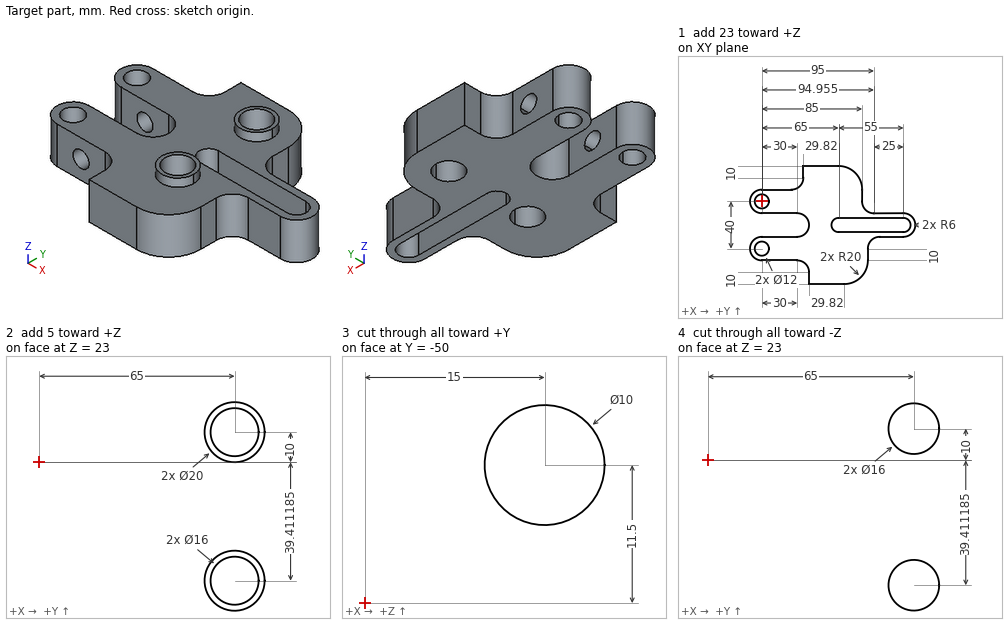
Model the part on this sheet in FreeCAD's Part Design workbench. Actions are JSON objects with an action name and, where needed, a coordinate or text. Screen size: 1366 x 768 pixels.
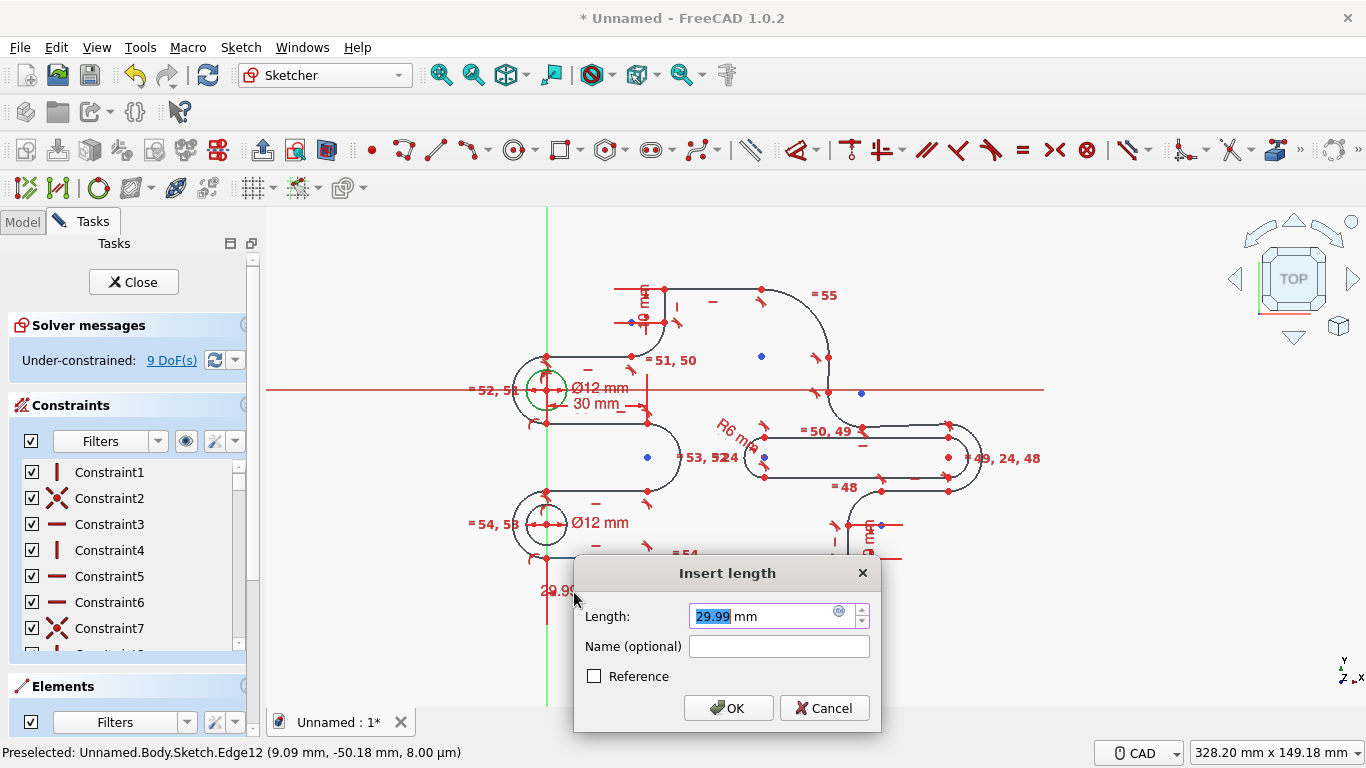
{"action": "type", "text": "30"}
{"action": "key", "text": "Return"}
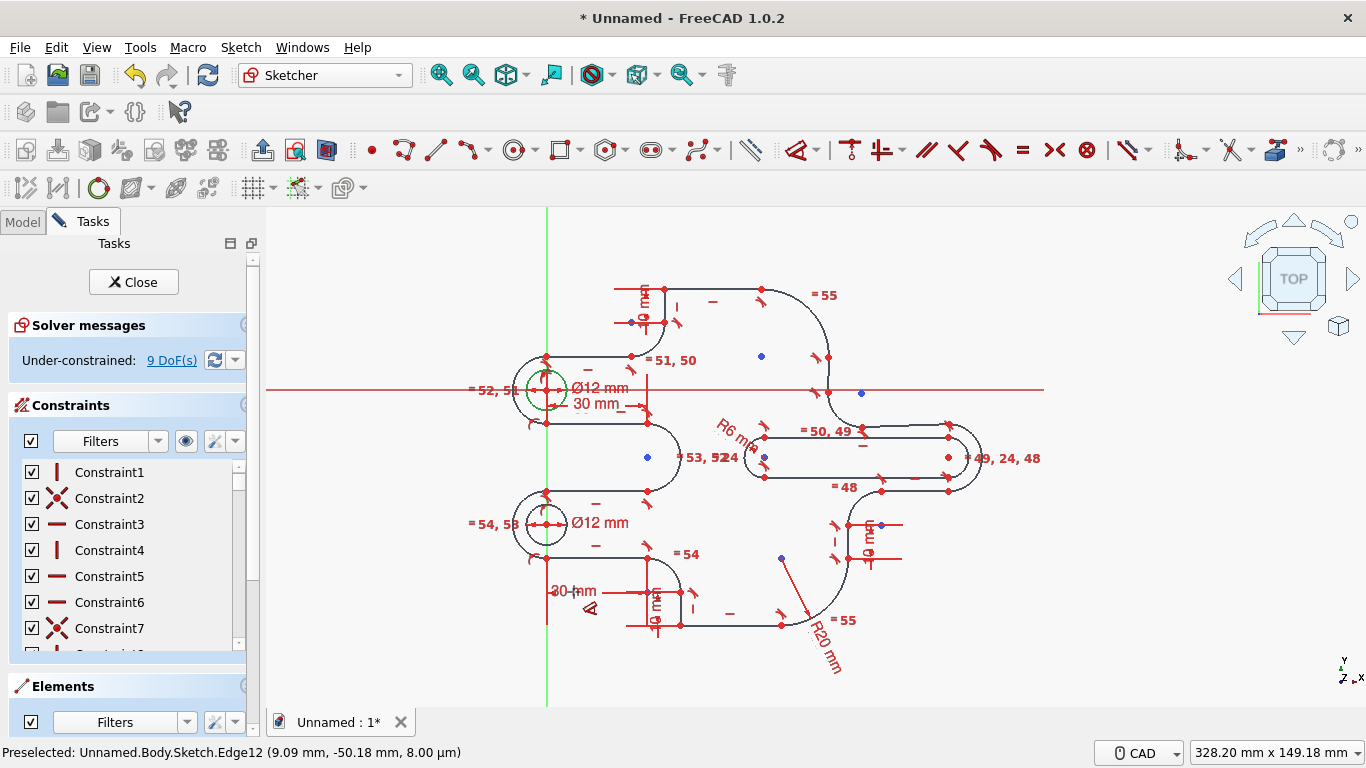
{"action": "left_click", "coordinate": [820, 438]}
{"action": "left_click", "coordinate": [856, 404]}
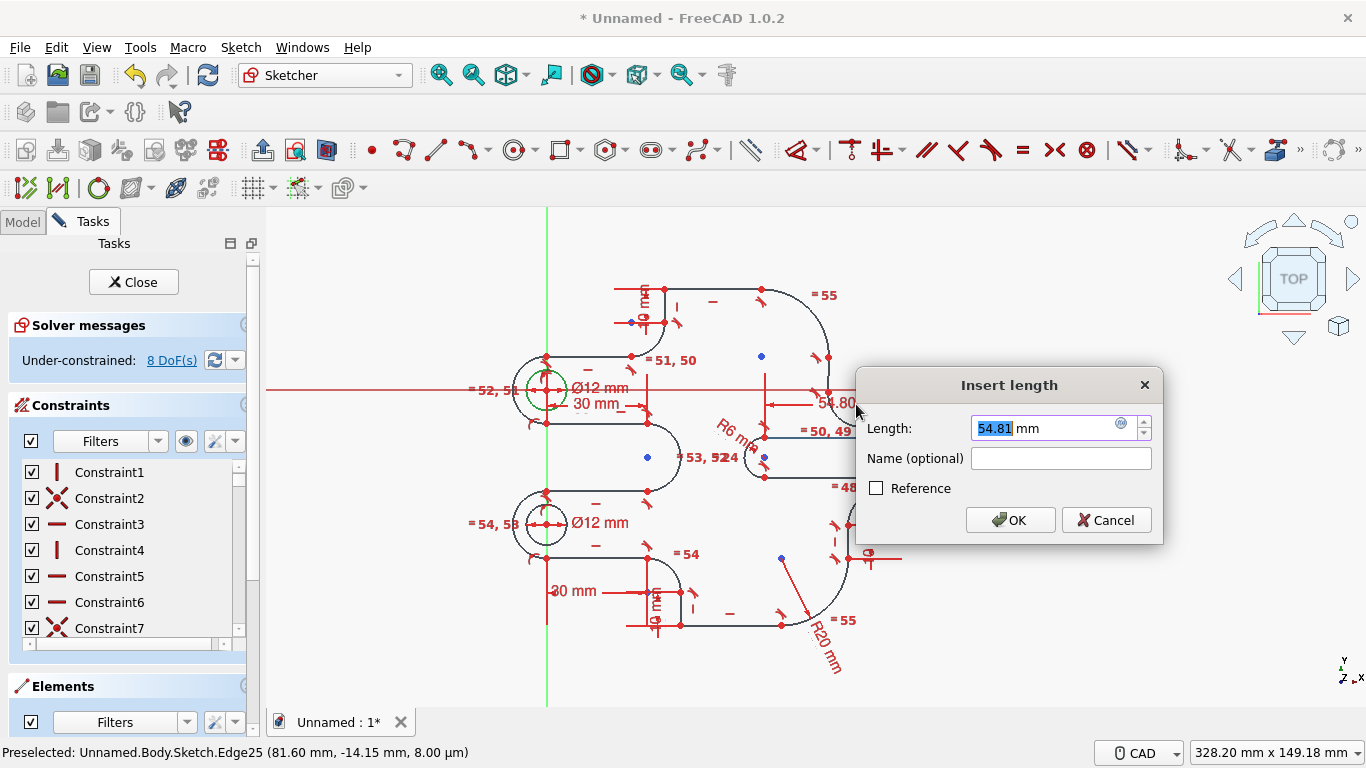
{"action": "type", "text": "55"}
{"action": "key", "text": "Return"}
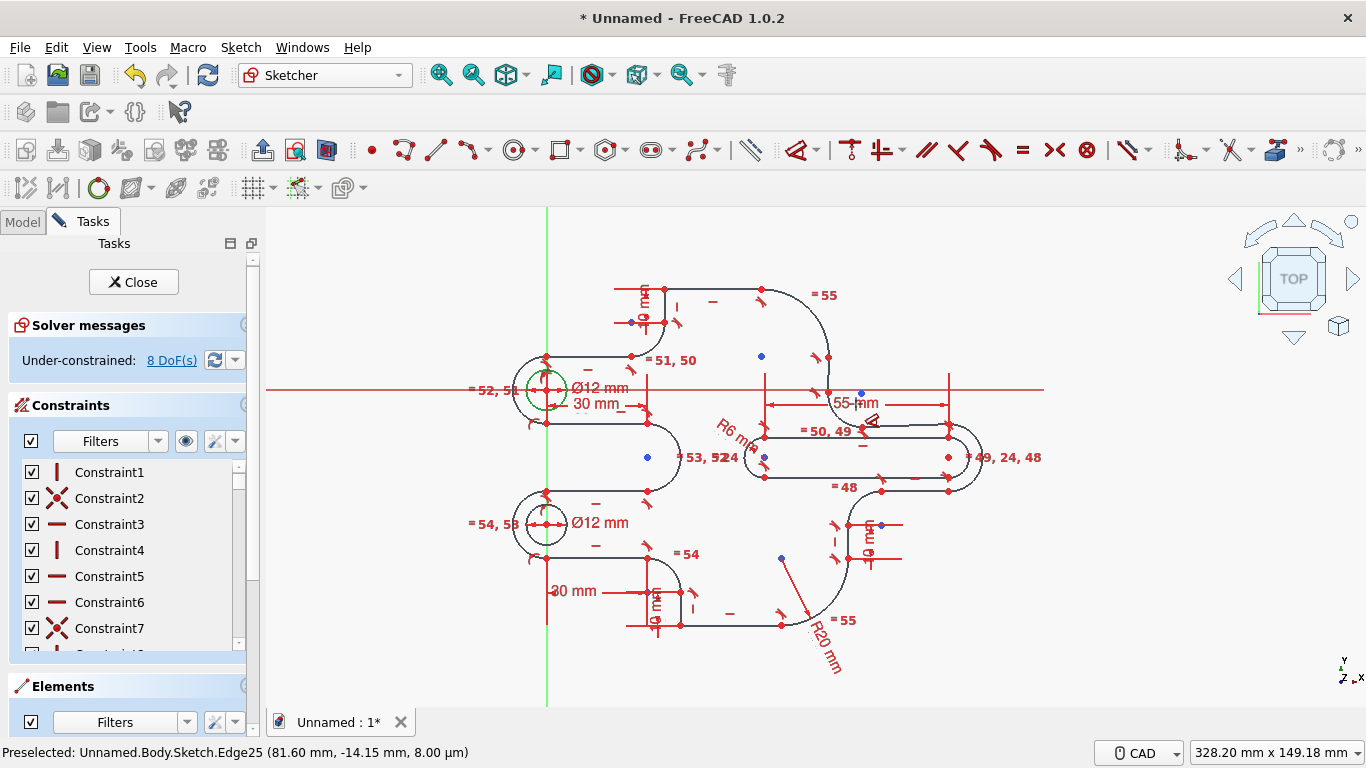
{"action": "left_click", "coordinate": [547, 525]}
{"action": "left_click", "coordinate": [513, 458]}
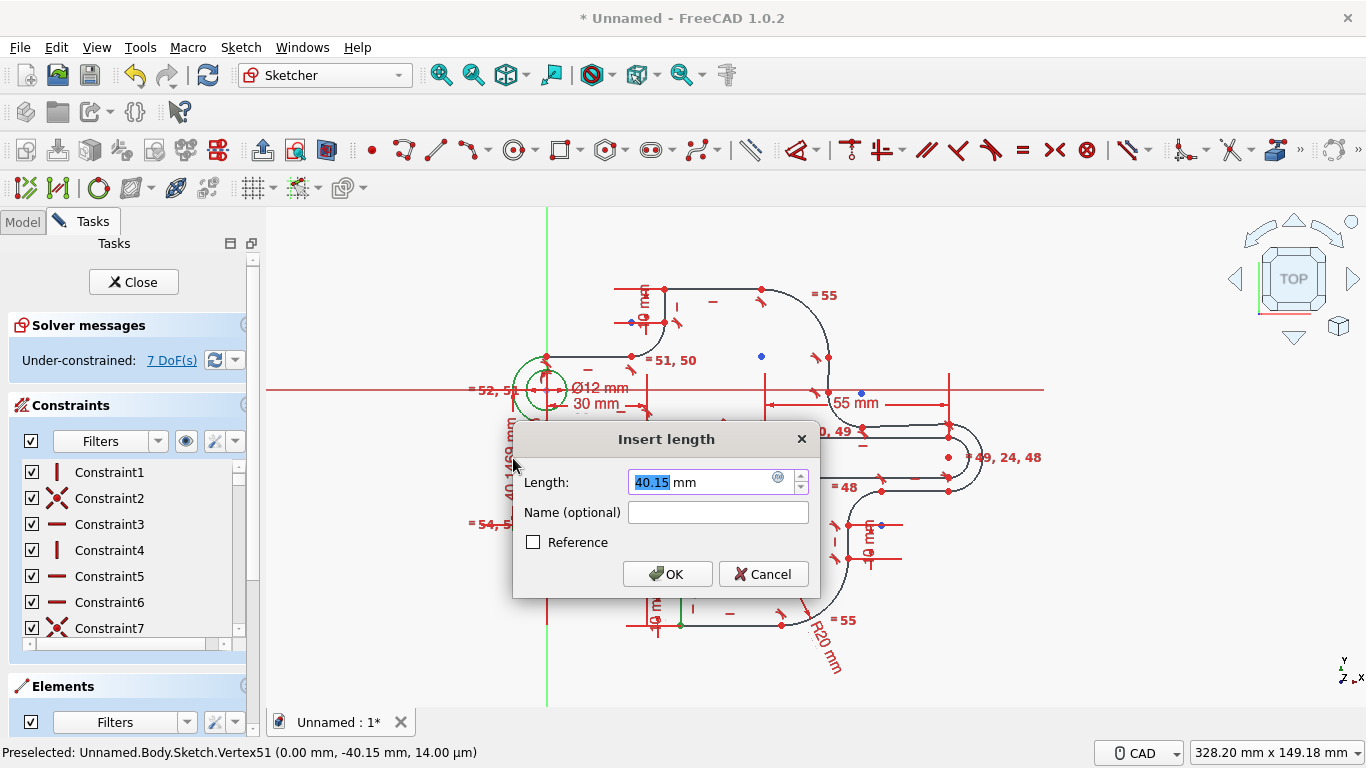
{"action": "type", "text": "40"}
{"action": "key", "text": "Return"}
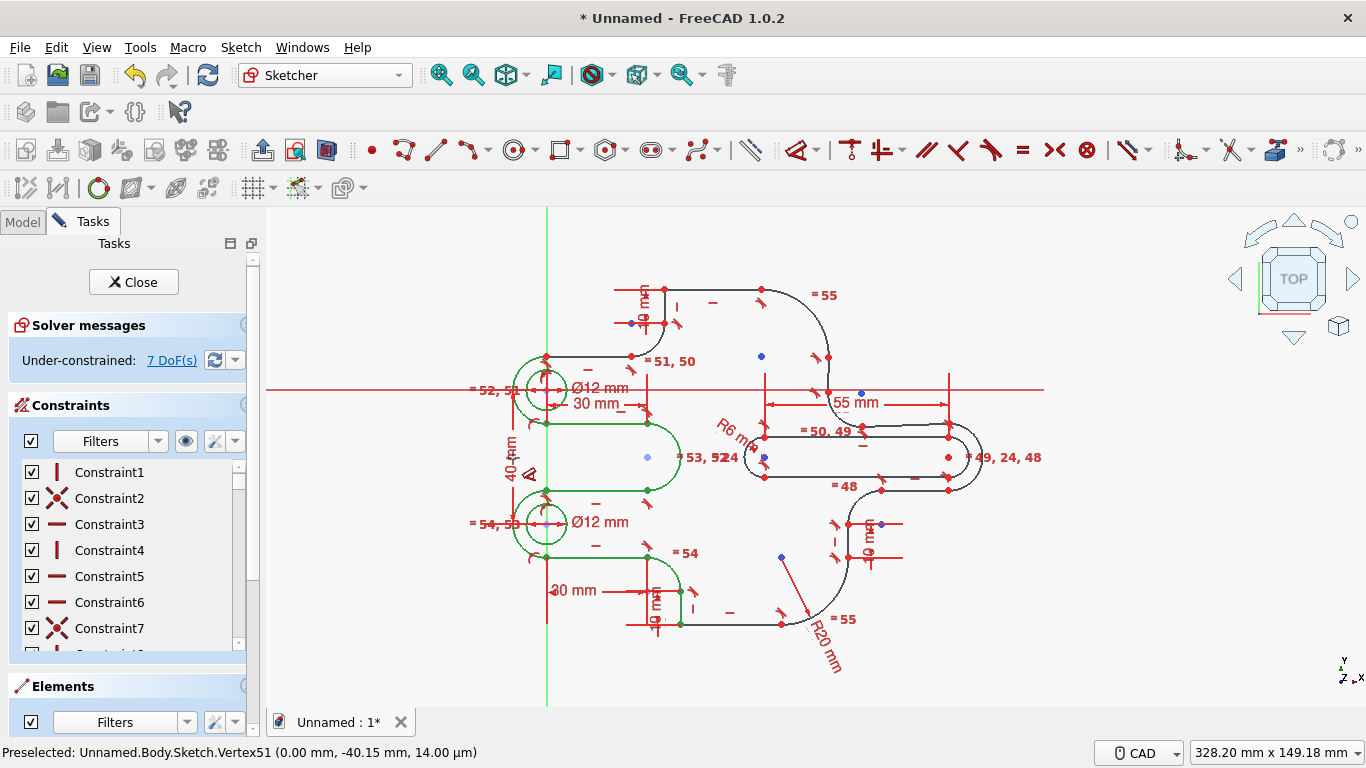
{"action": "left_click", "coordinate": [863, 427]}
{"action": "left_click", "coordinate": [705, 356]}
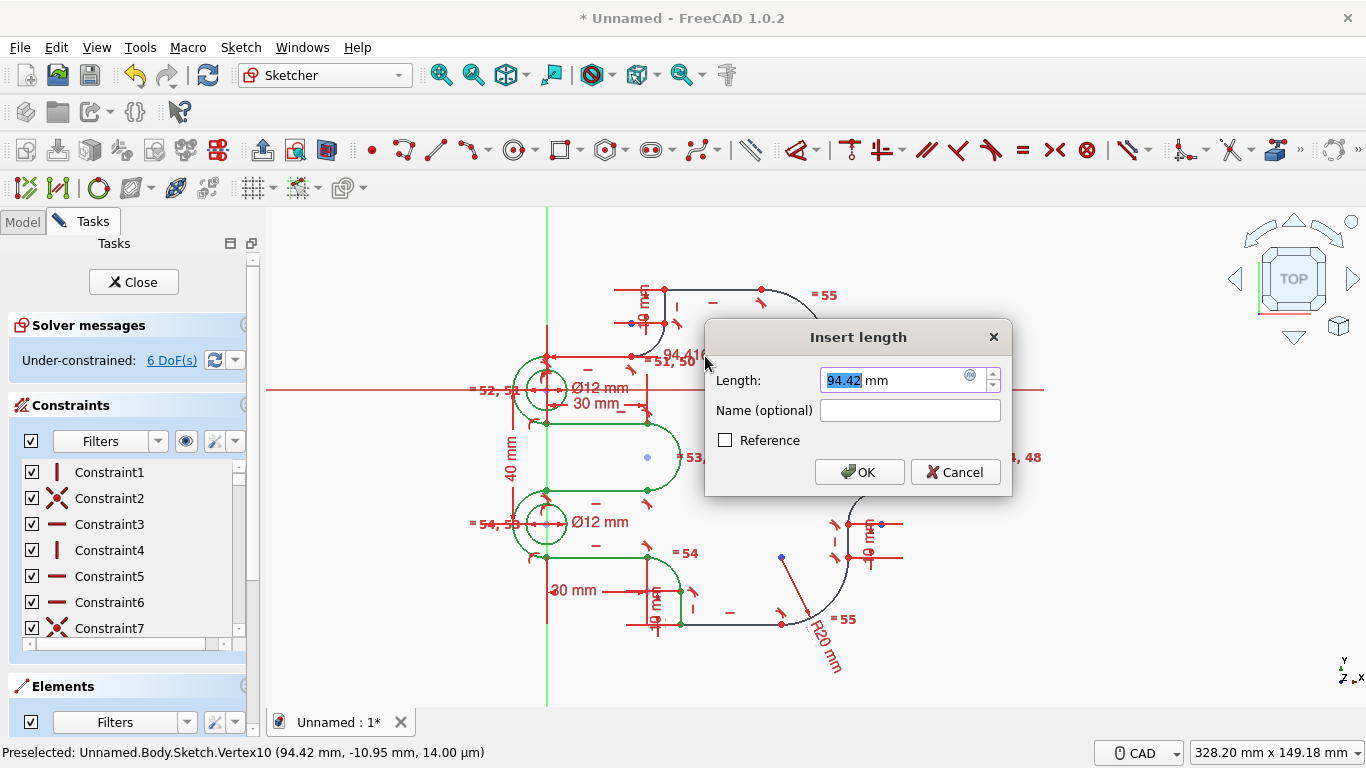
{"action": "type", "text": "95"}
{"action": "key", "text": "Return"}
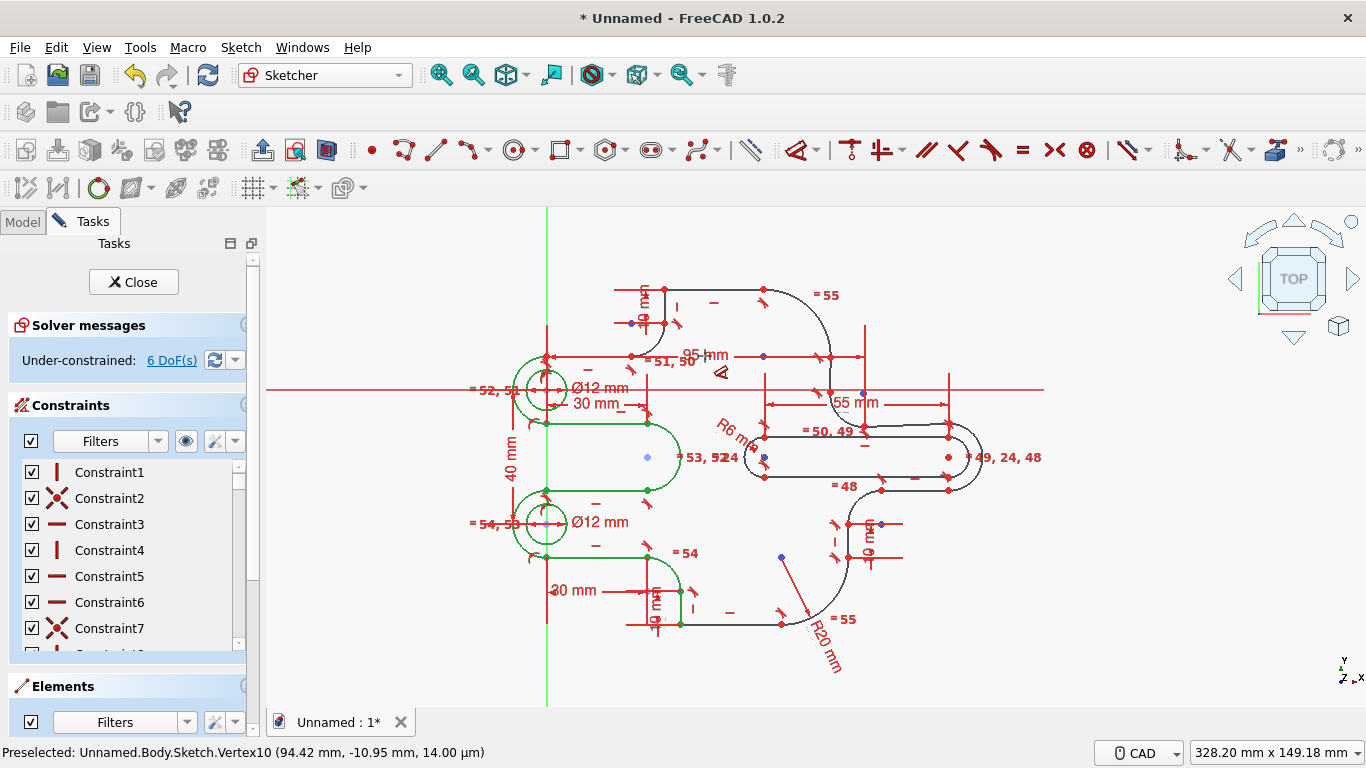
{"action": "left_click", "coordinate": [831, 358]}
{"action": "left_click", "coordinate": [754, 324]}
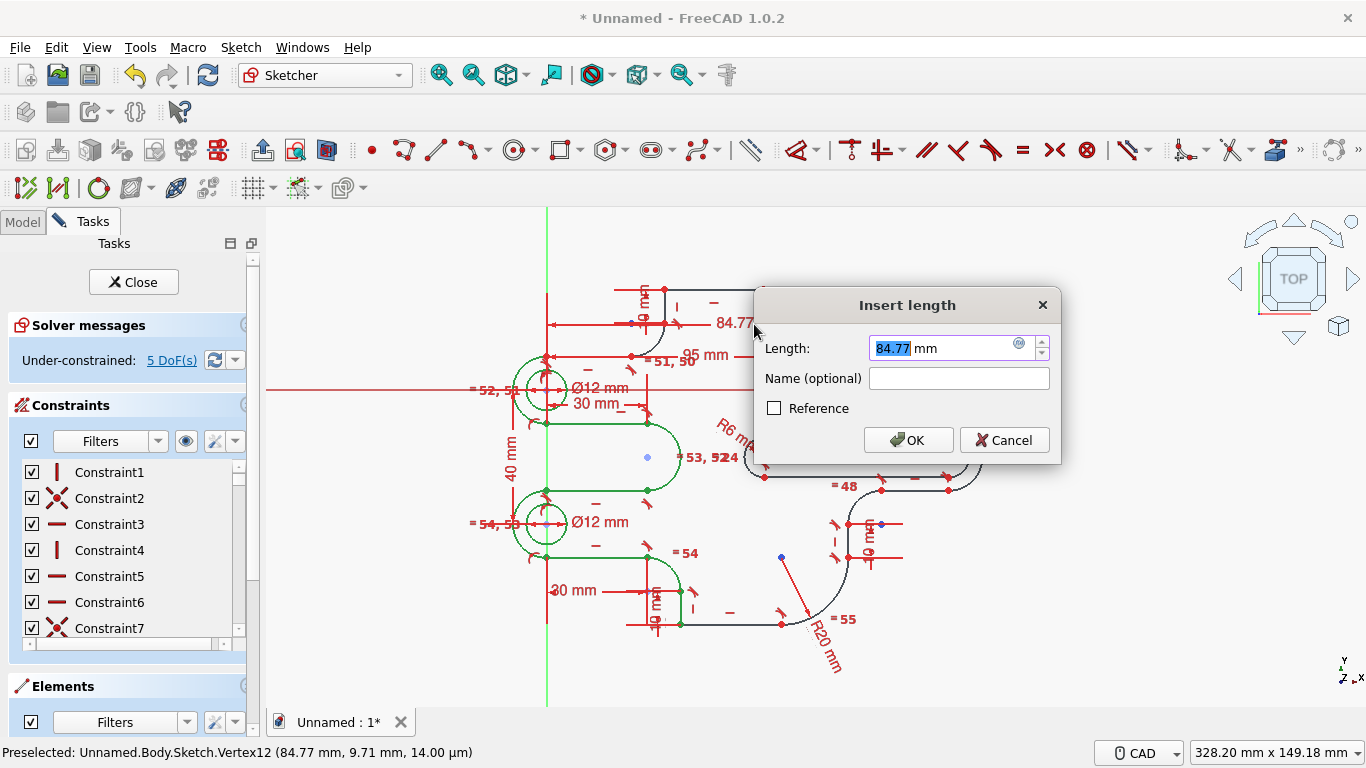
{"action": "type", "text": "85"}
{"action": "key", "text": "Return"}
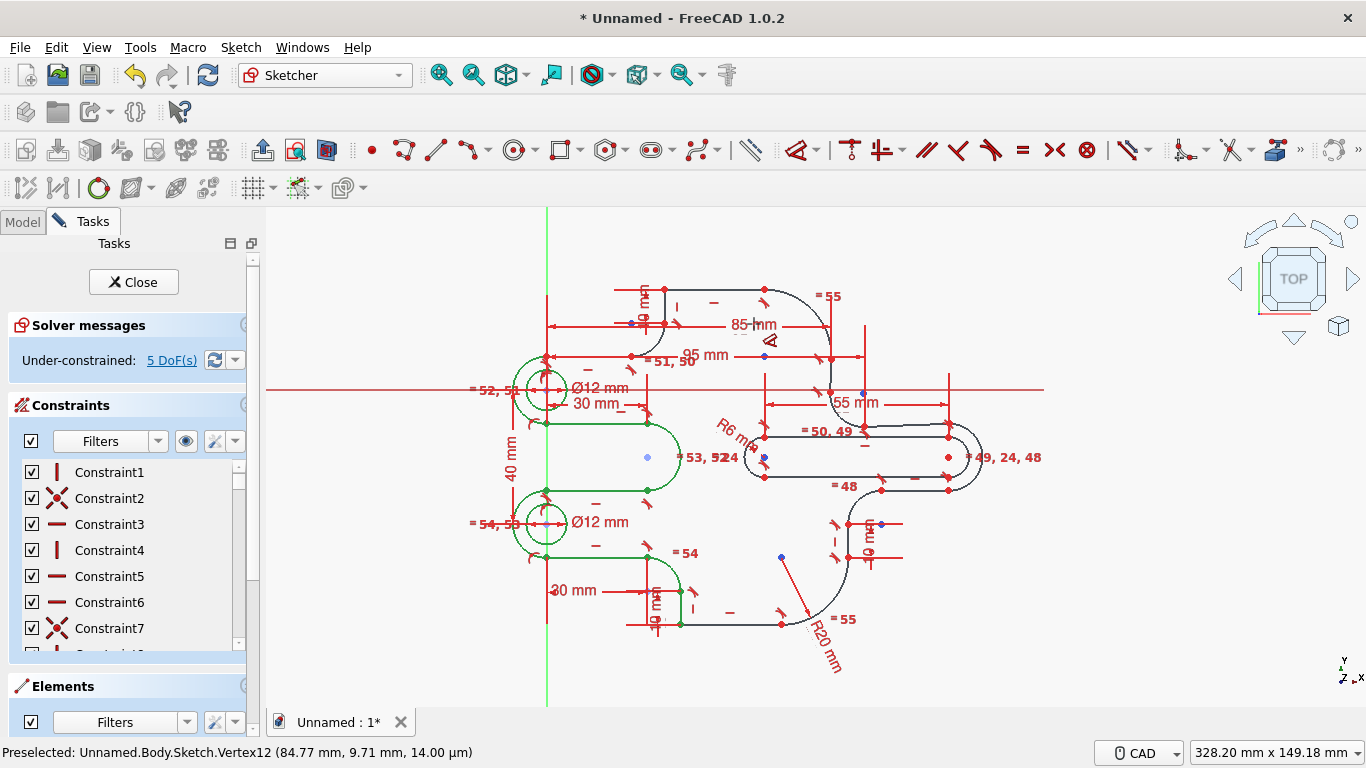
{"action": "left_click", "coordinate": [765, 437]}
{"action": "left_click", "coordinate": [656, 471]}